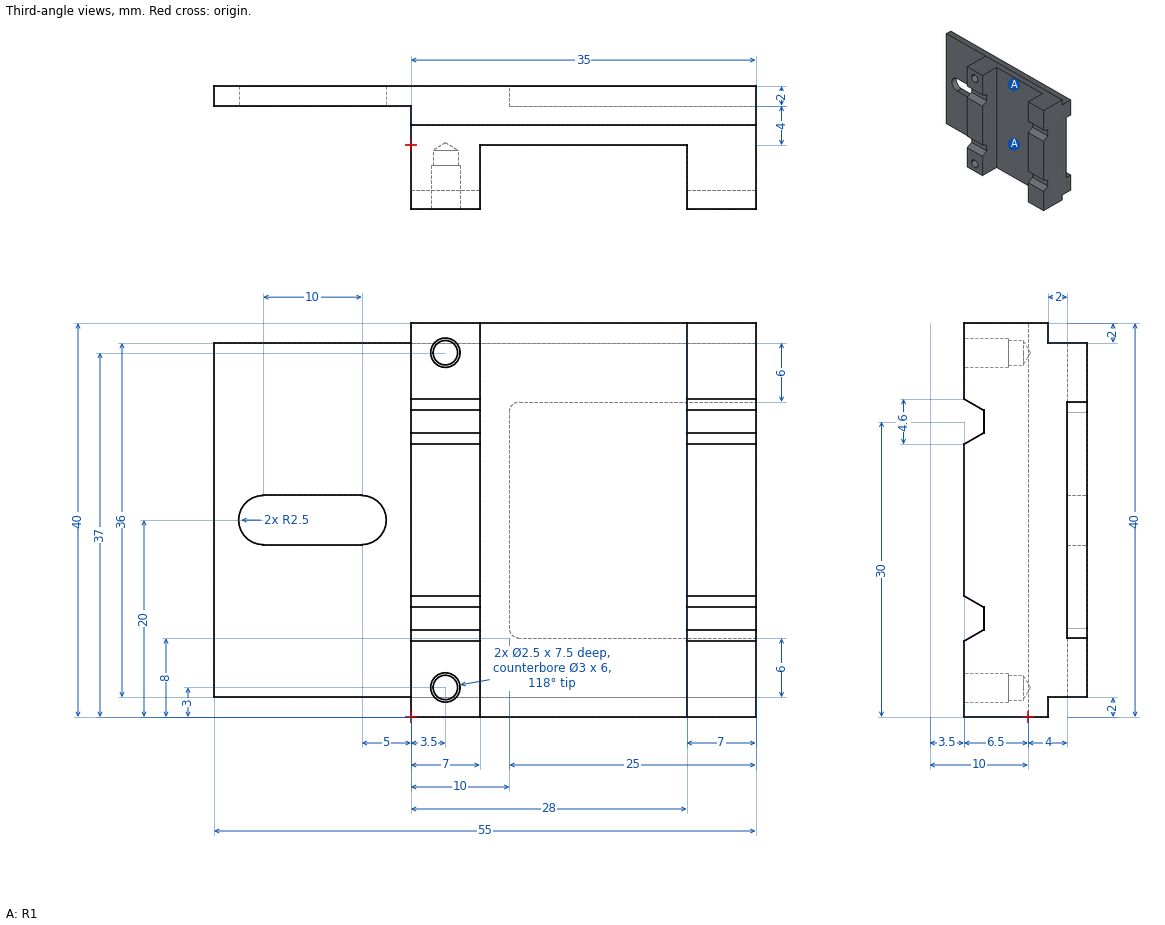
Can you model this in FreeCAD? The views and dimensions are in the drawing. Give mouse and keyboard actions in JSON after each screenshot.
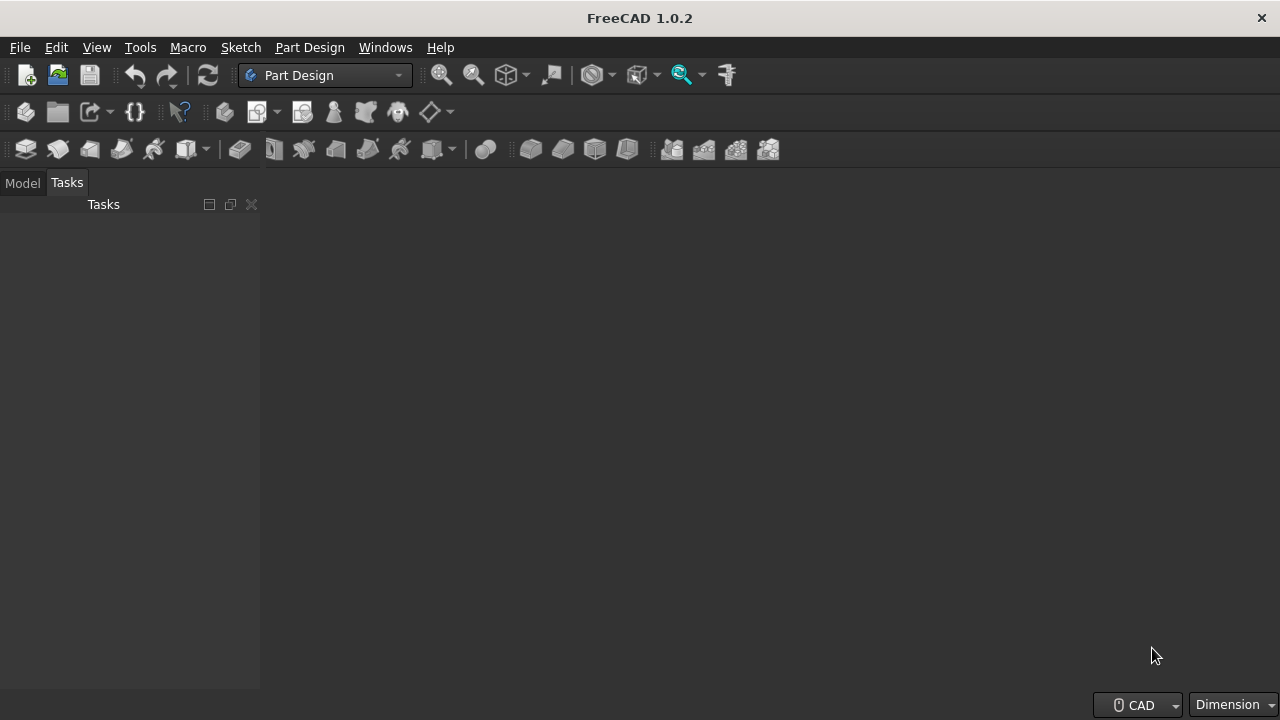
{"action": "left_click", "coordinate": [26, 76]}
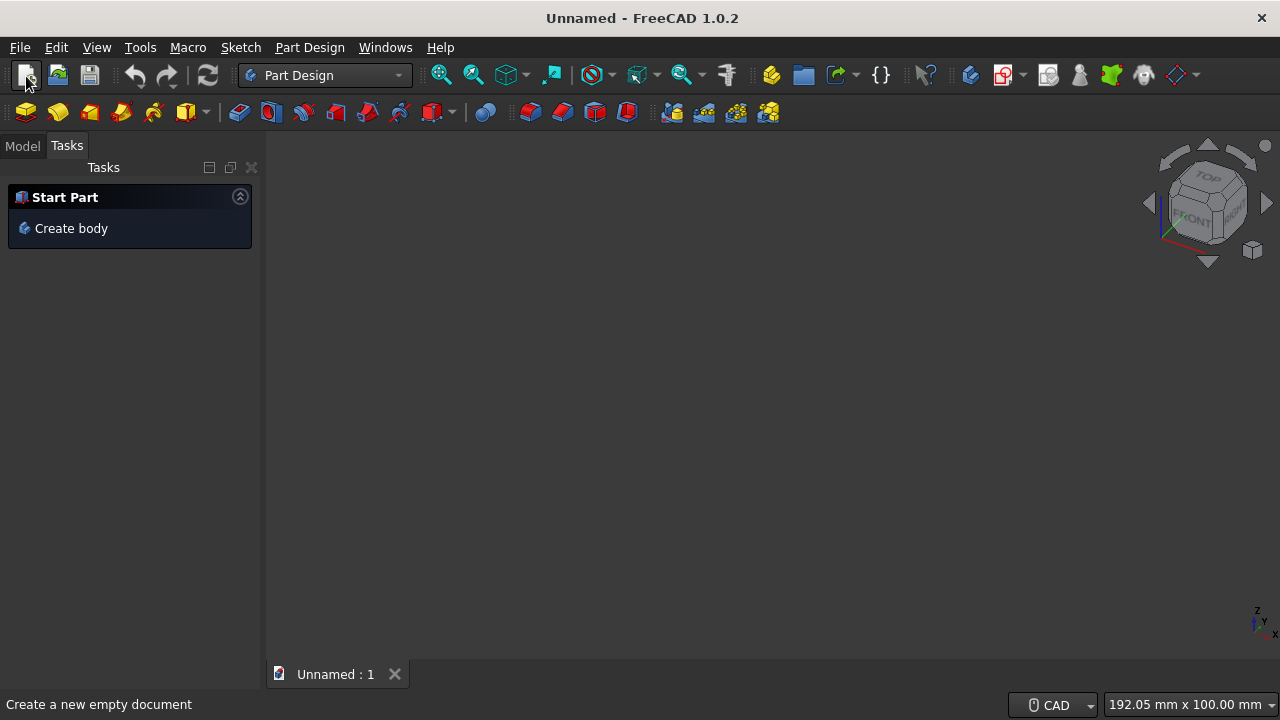
{"action": "left_click", "coordinate": [1004, 76]}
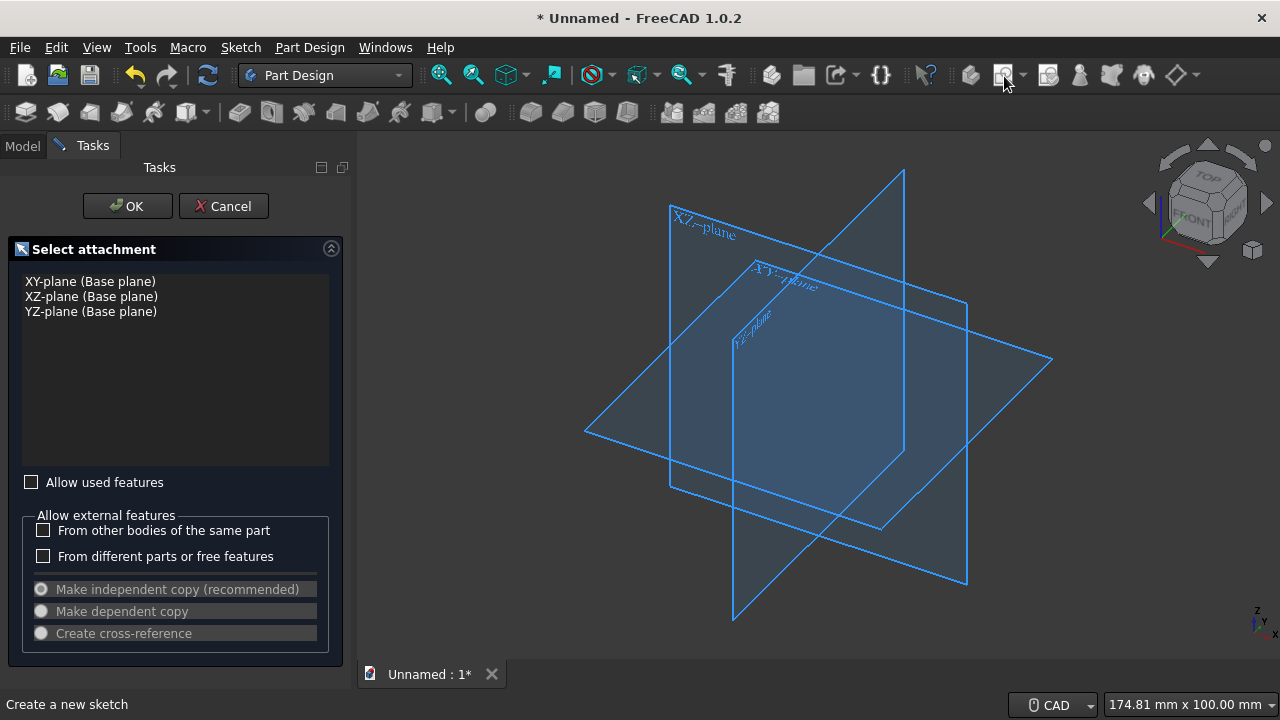
{"action": "left_click", "coordinate": [82, 282]}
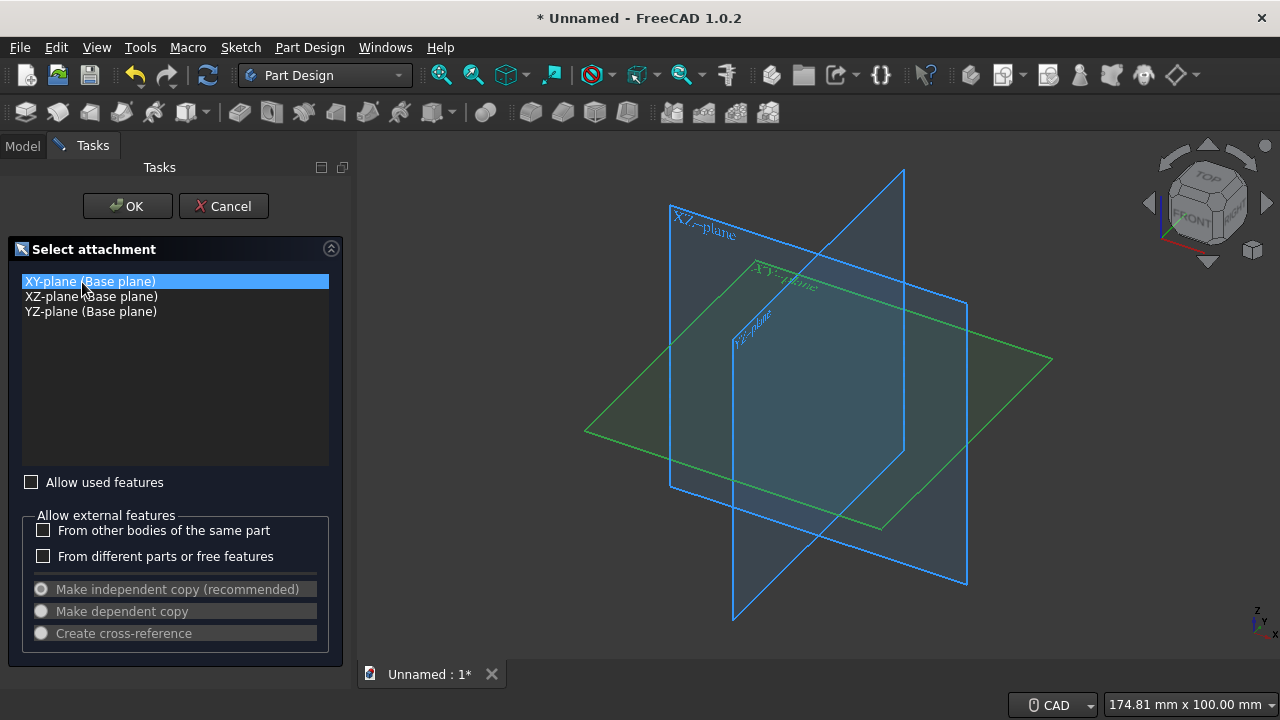
{"action": "left_click", "coordinate": [128, 206]}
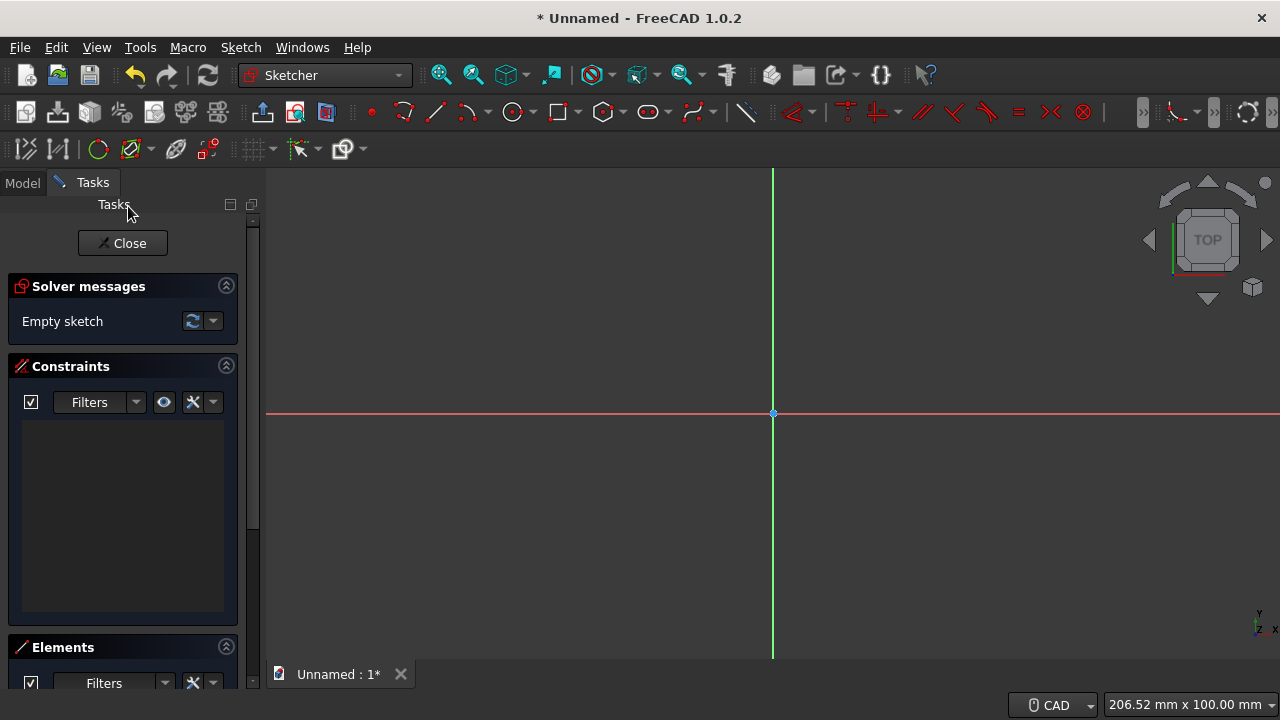
{"action": "scroll", "coordinate": [925, 399], "scroll_direction": "up", "scroll_amount": 6}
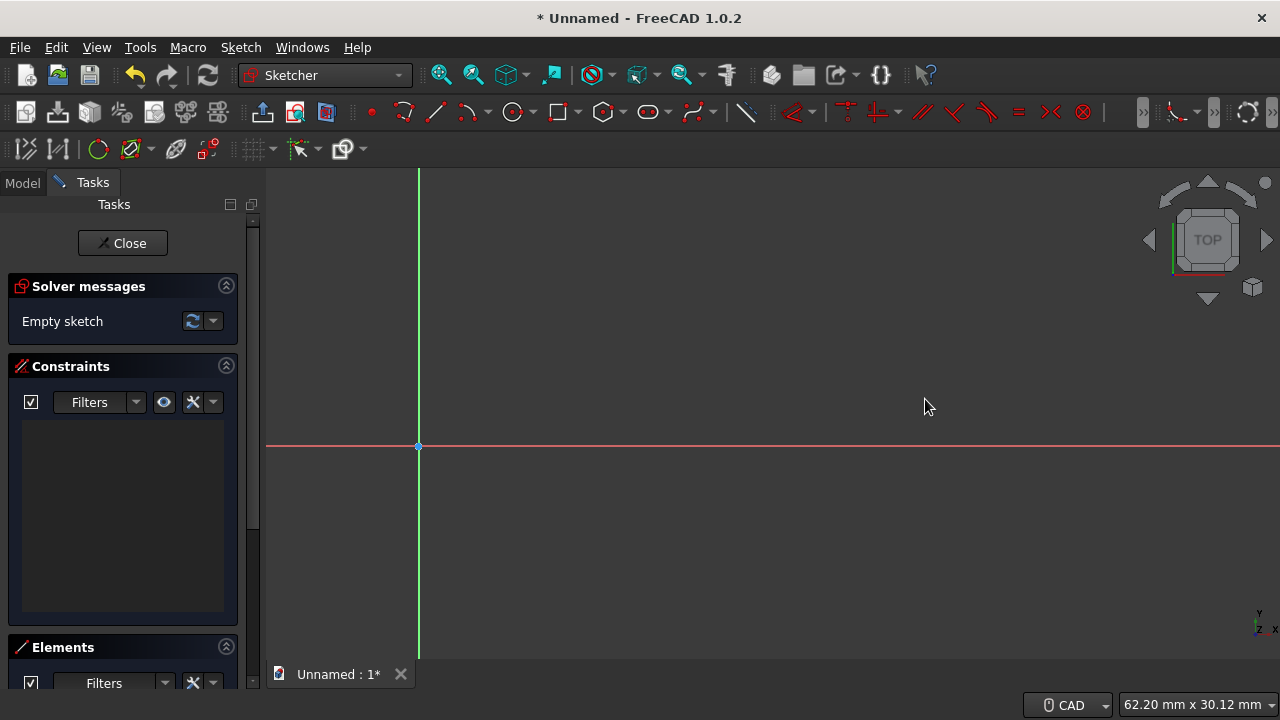
{"action": "left_click", "coordinate": [558, 112]}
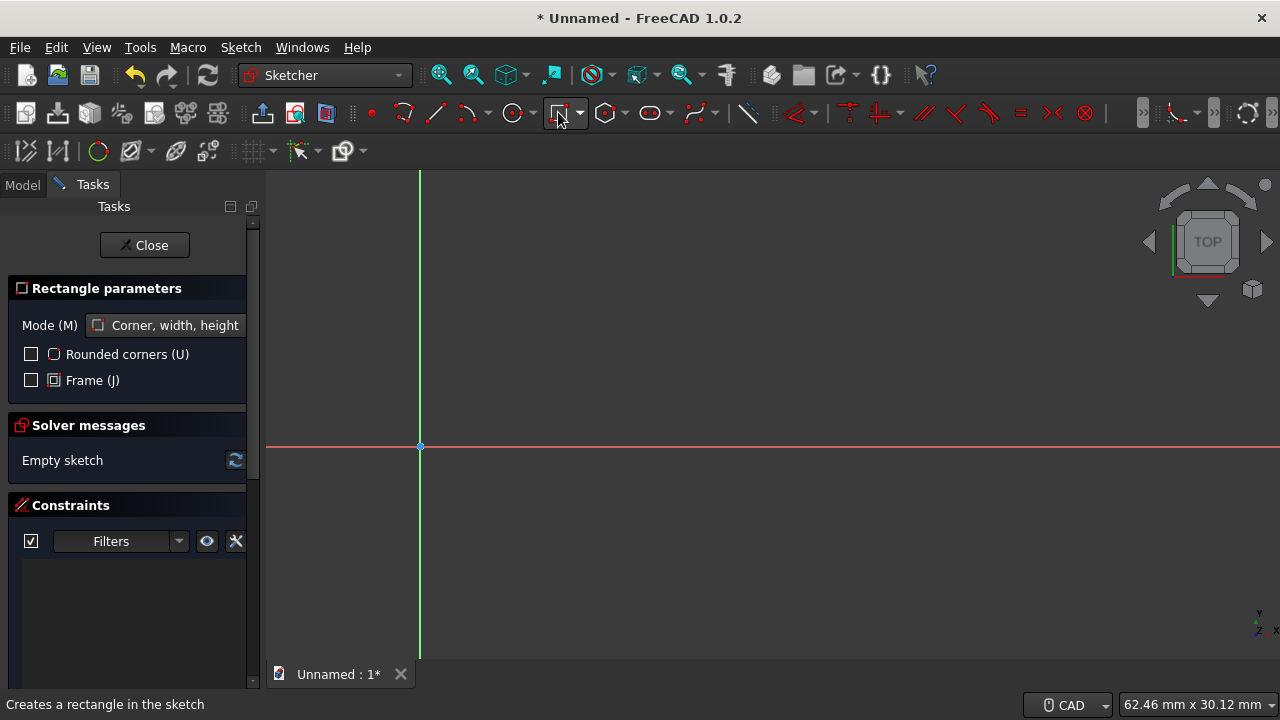
{"action": "left_click", "coordinate": [420, 447]}
{"action": "mouse_move", "coordinate": [989, 382]}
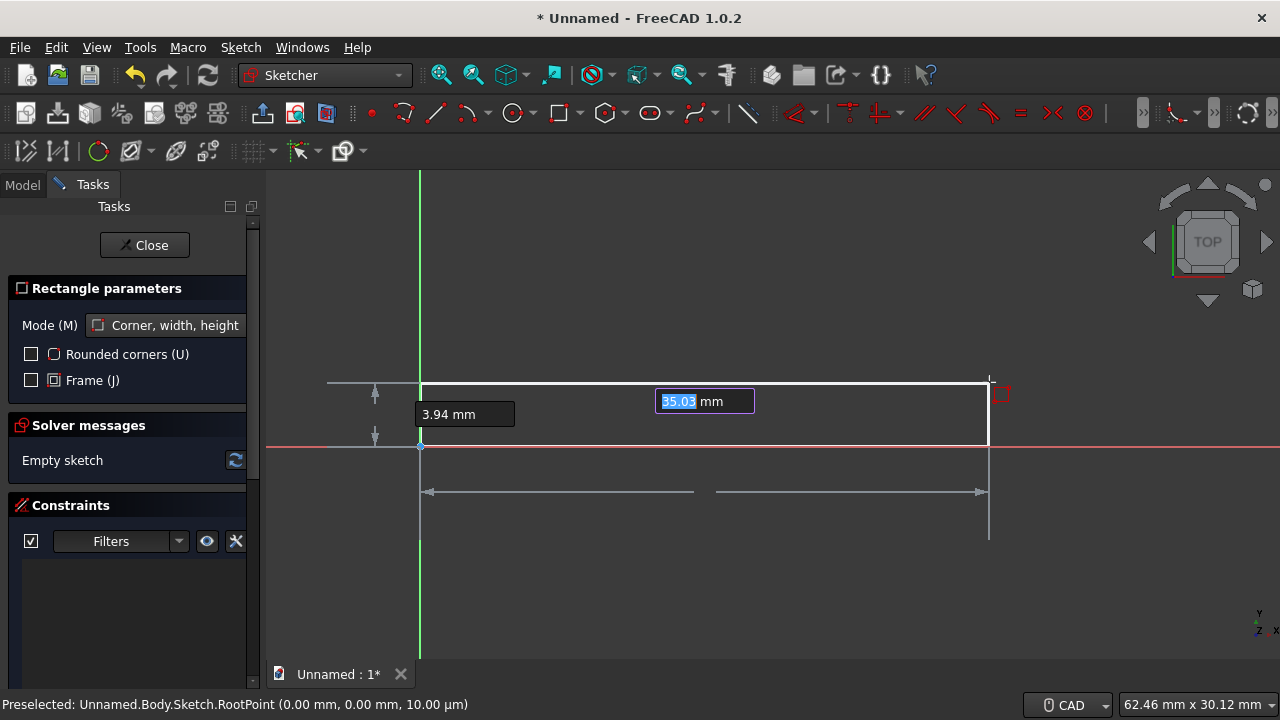
{"action": "type", "text": "35"}
{"action": "key", "text": "Tab"}
{"action": "type", "text": "4"}
{"action": "key", "text": "Return"}
{"action": "key", "text": "Escape"}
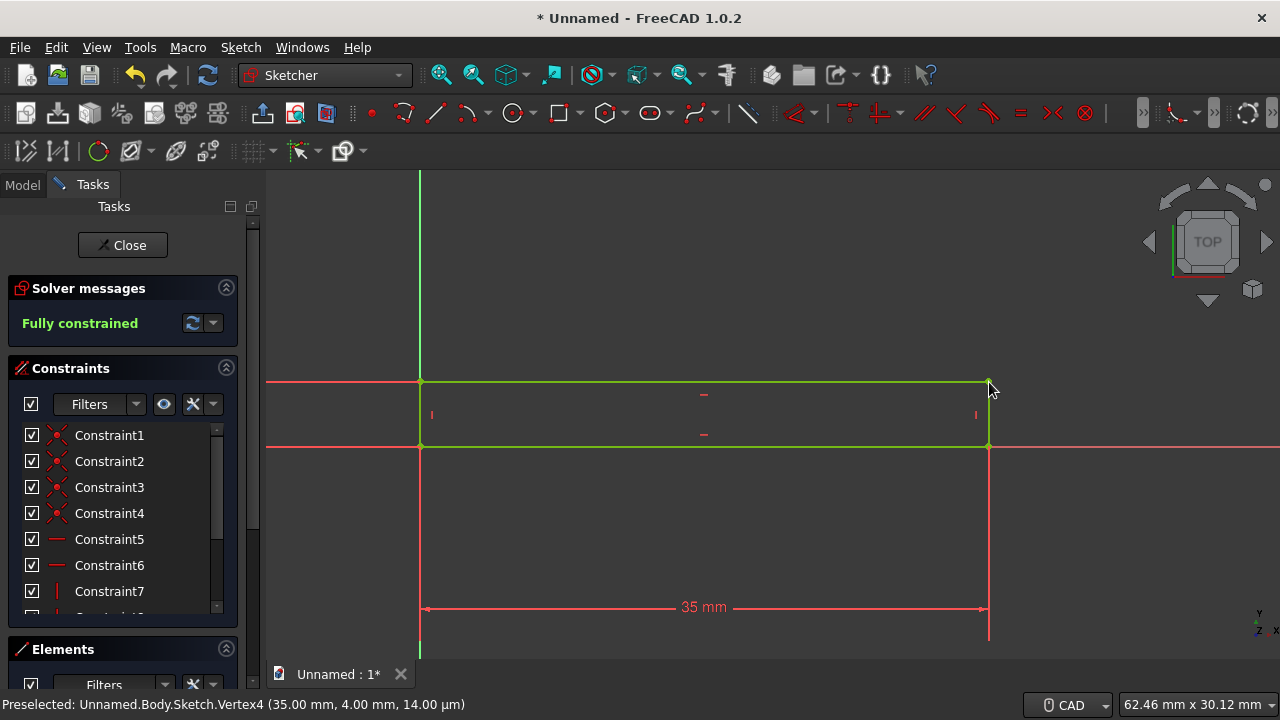
{"action": "left_click", "coordinate": [123, 245]}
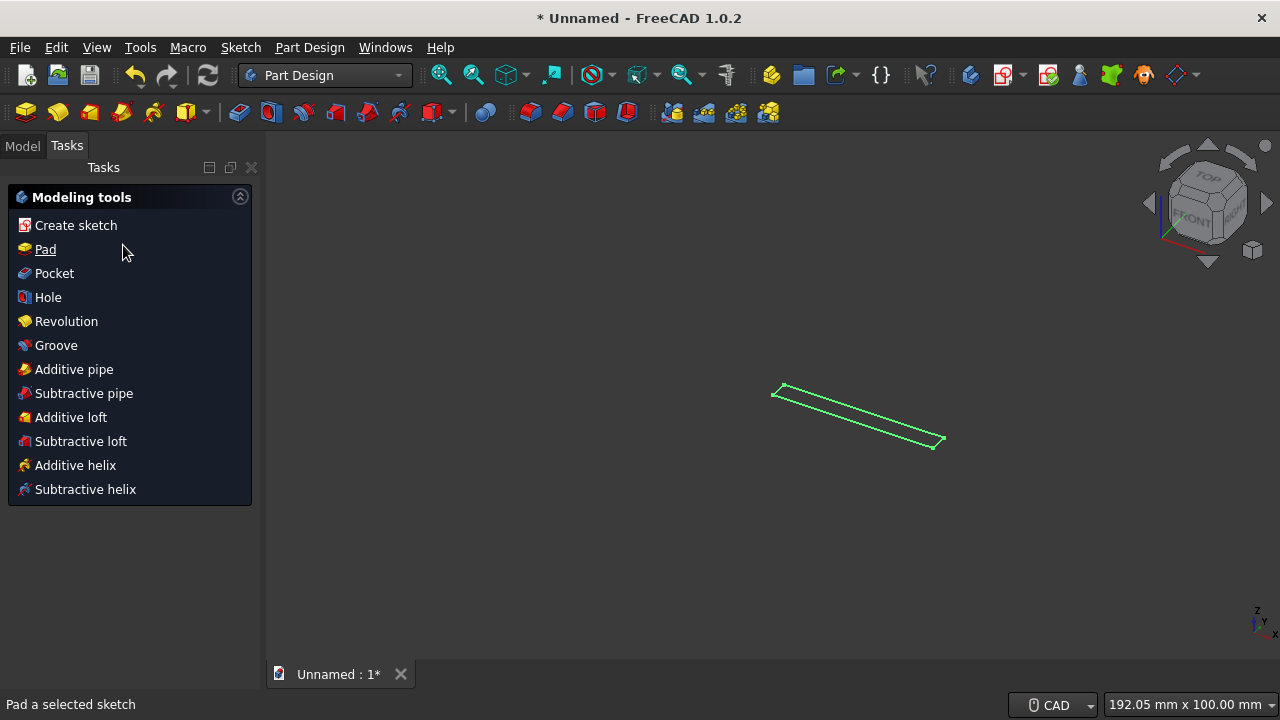
{"action": "left_click", "coordinate": [26, 112]}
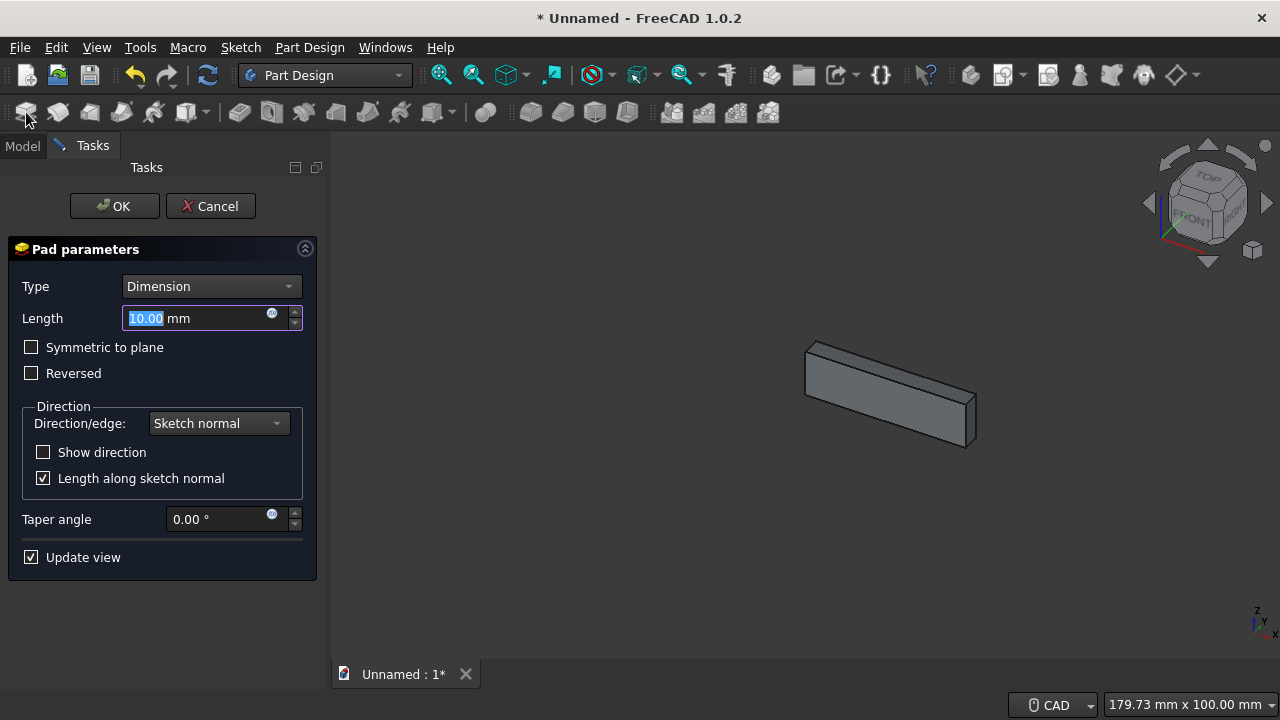
{"action": "type", "text": "40"}
{"action": "key", "text": "Tab"}